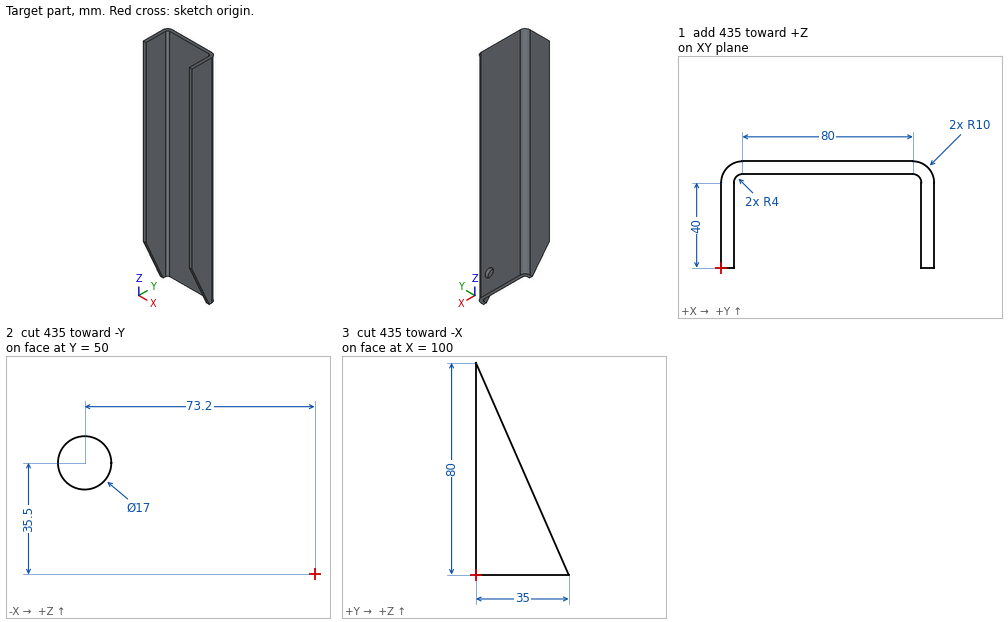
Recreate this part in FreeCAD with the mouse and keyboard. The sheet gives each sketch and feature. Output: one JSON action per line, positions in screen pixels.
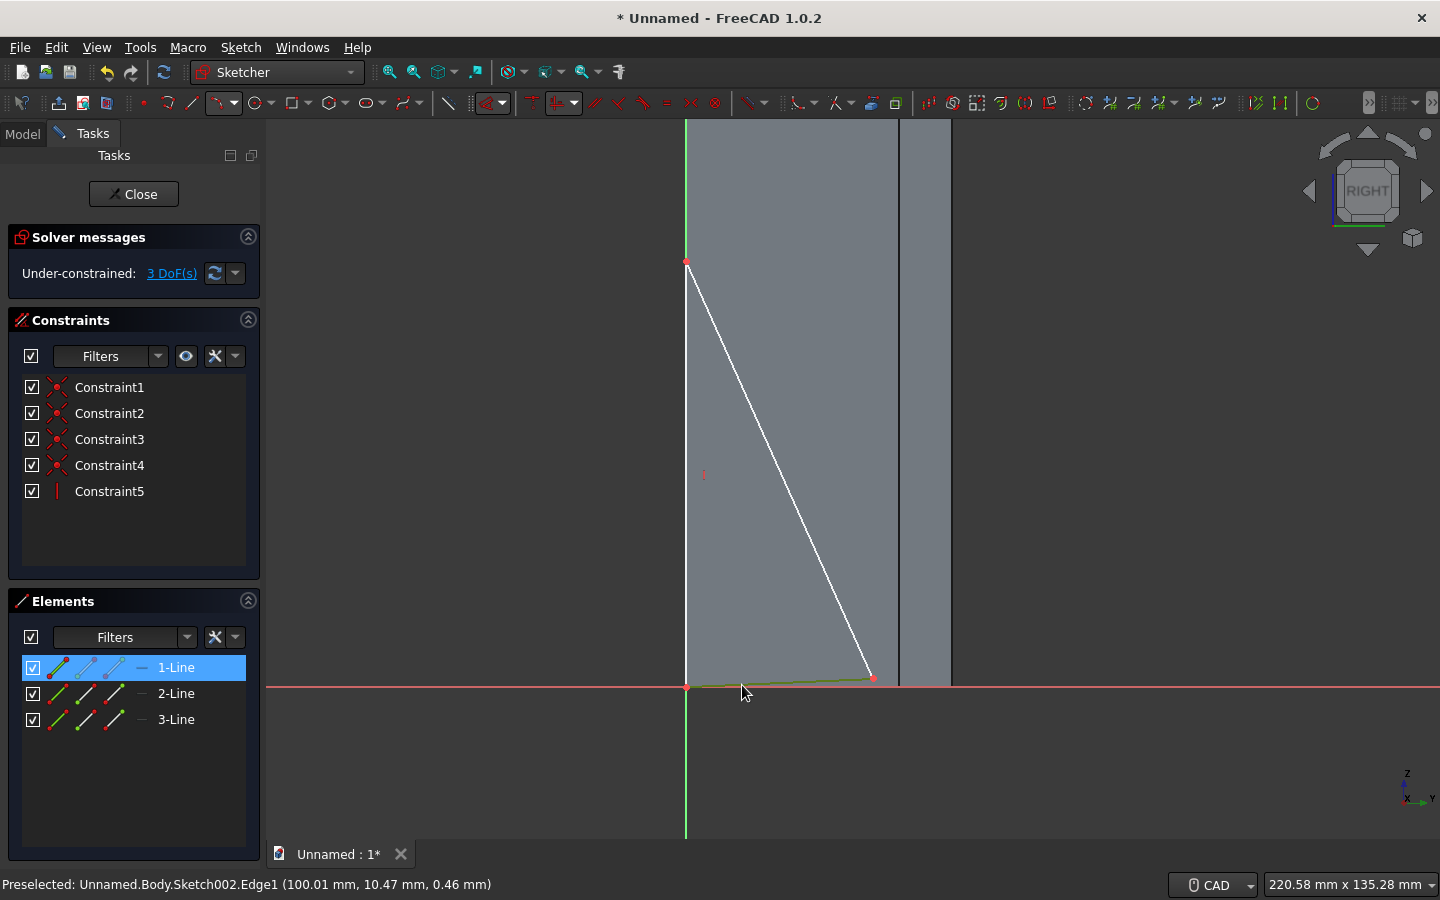
{"action": "key", "text": "h"}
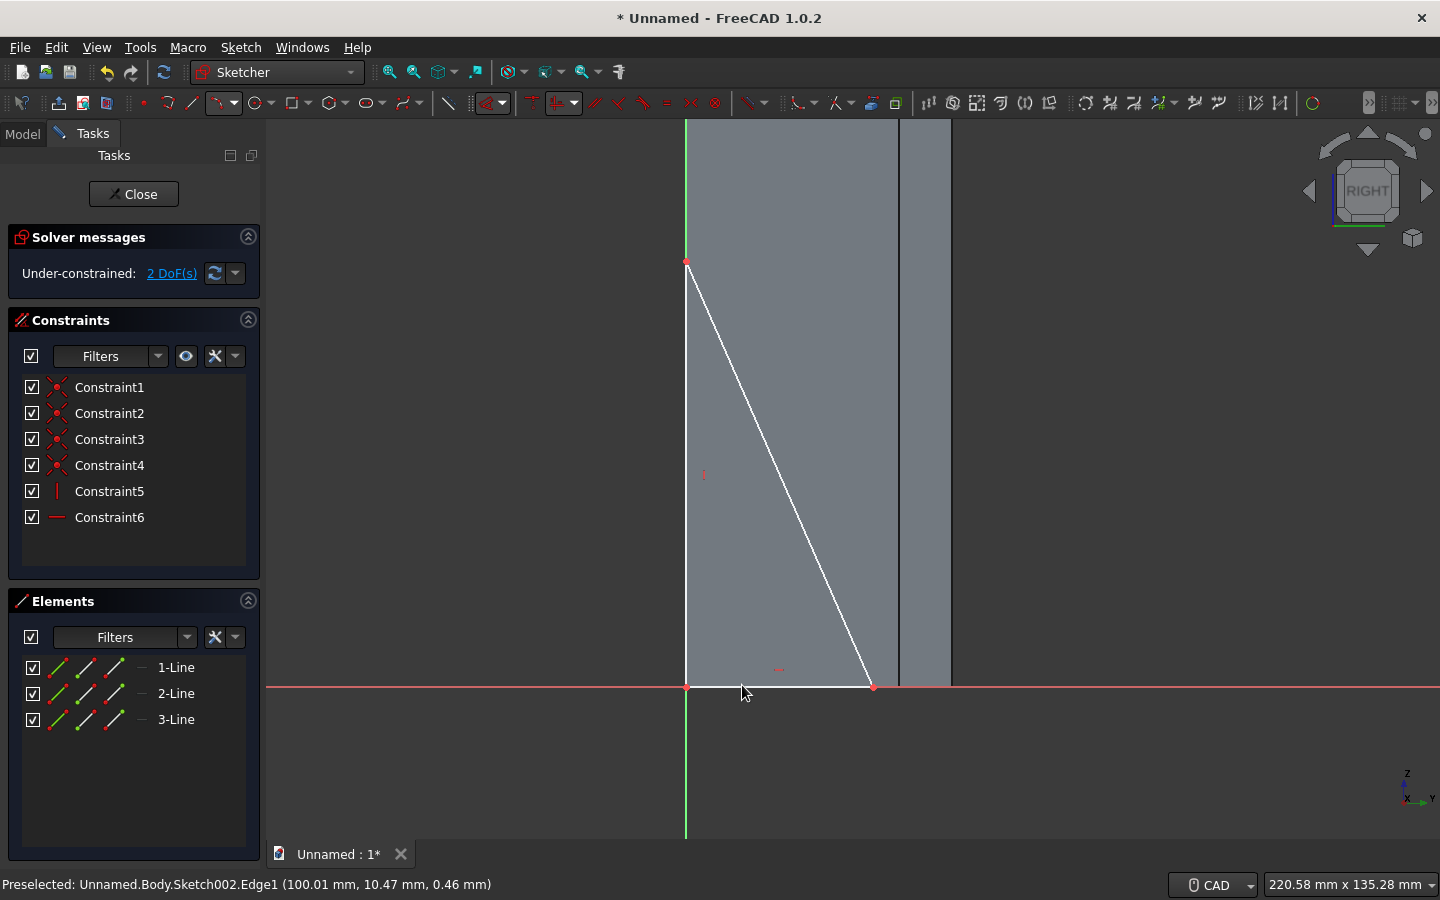
{"action": "left_click", "coordinate": [742, 687]}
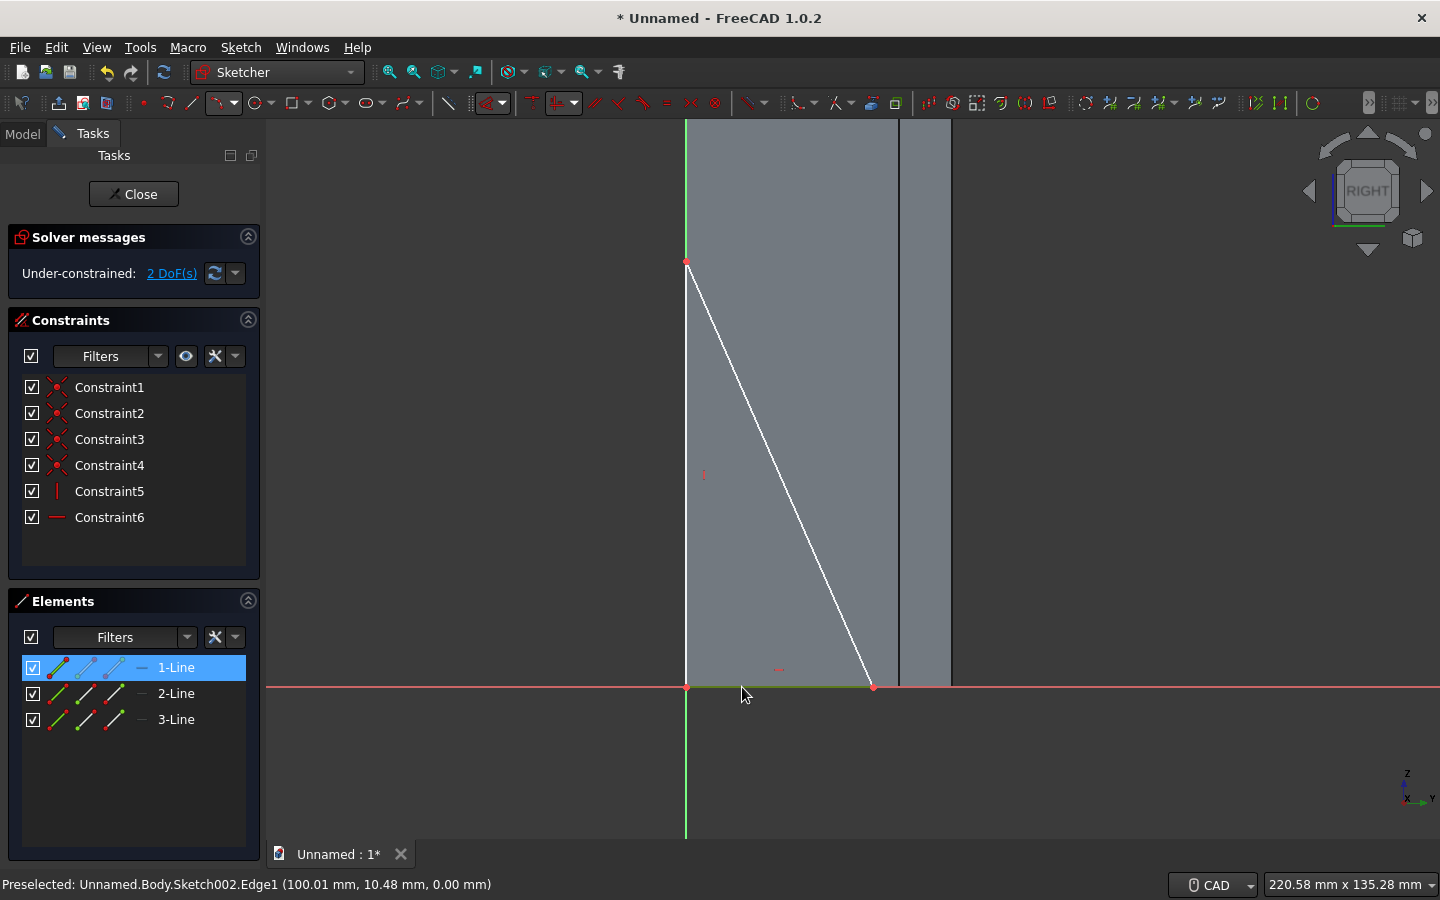
{"action": "key", "text": "l"}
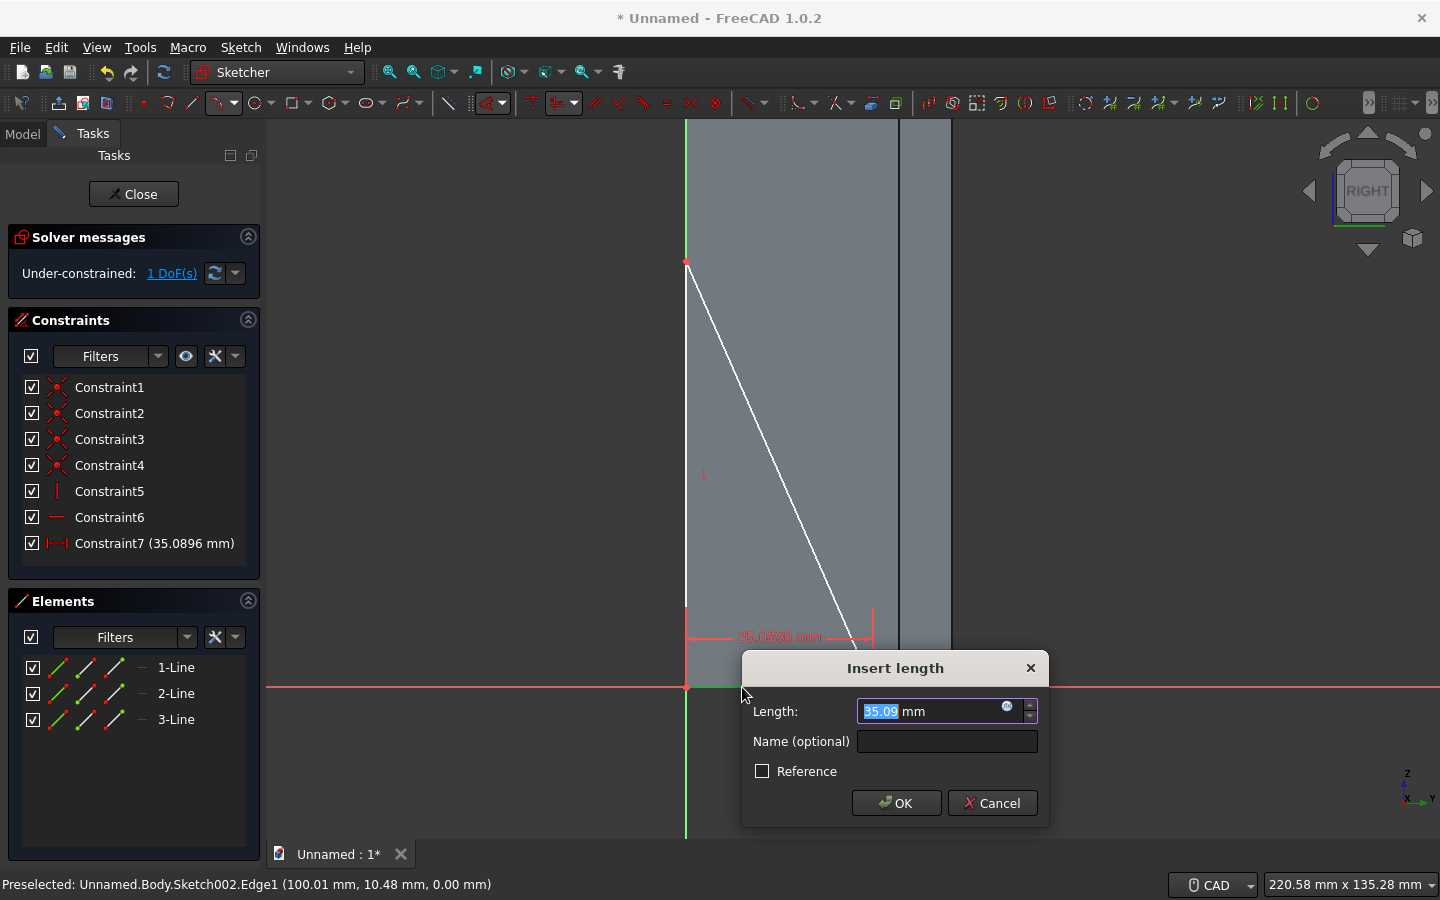
{"action": "type", "text": "35"}
{"action": "key", "text": "Return"}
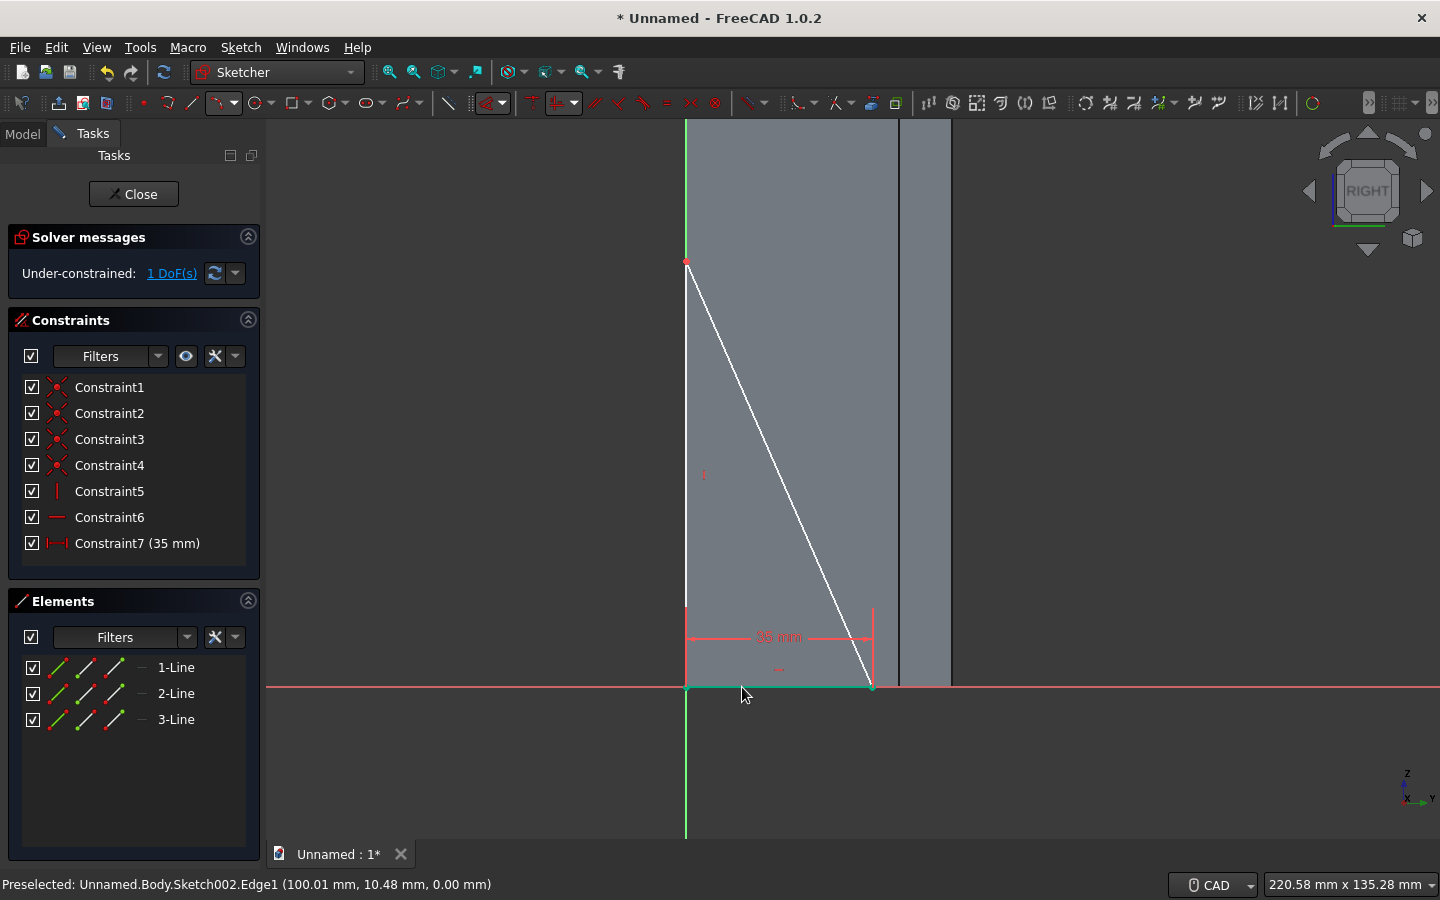
{"action": "left_click", "coordinate": [686, 390]}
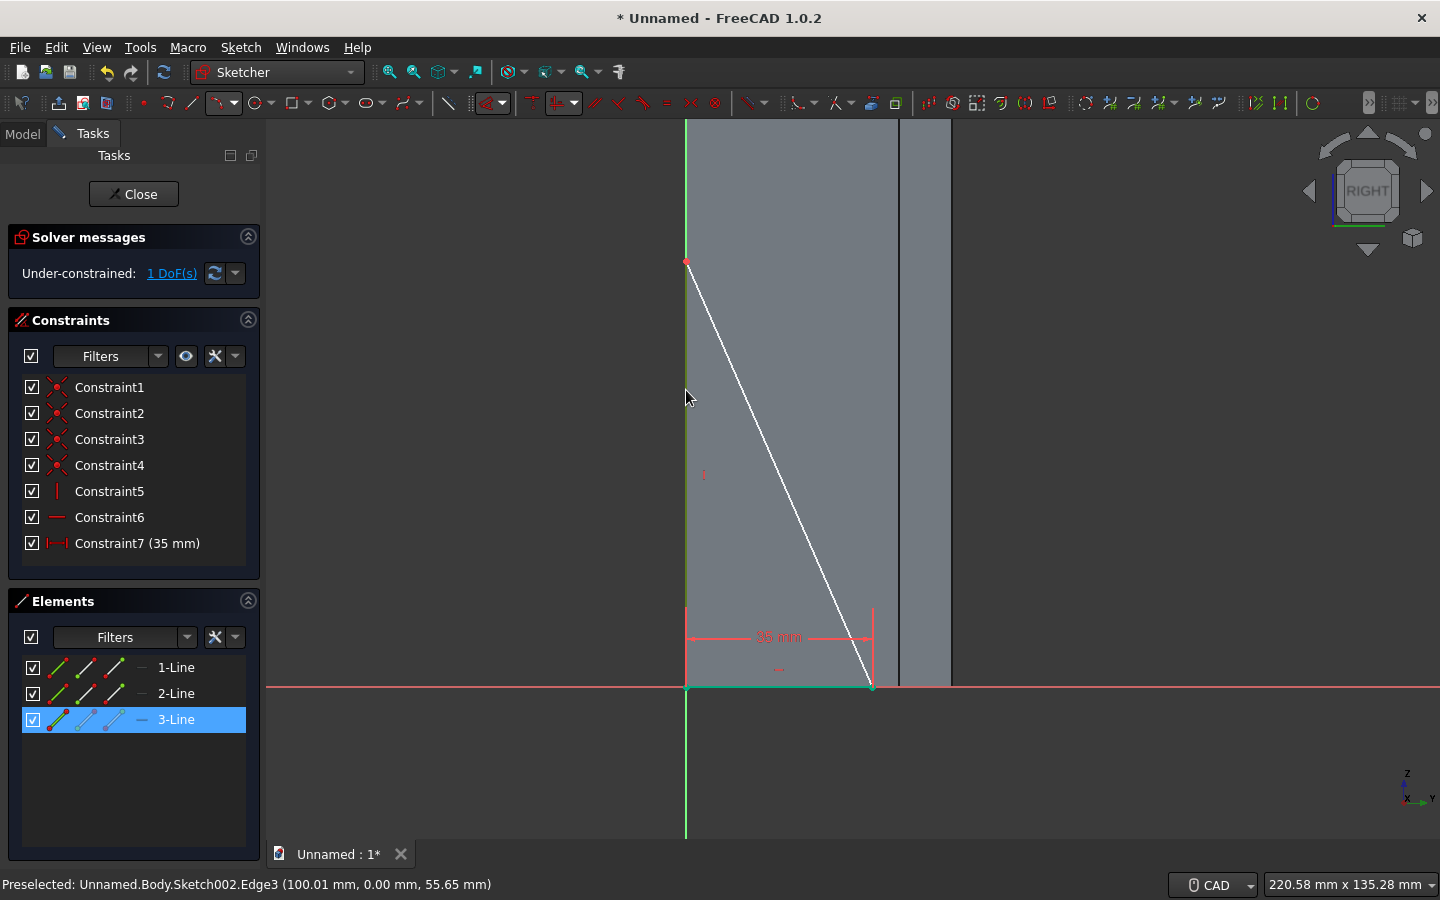
{"action": "left_click", "coordinate": [504, 104]}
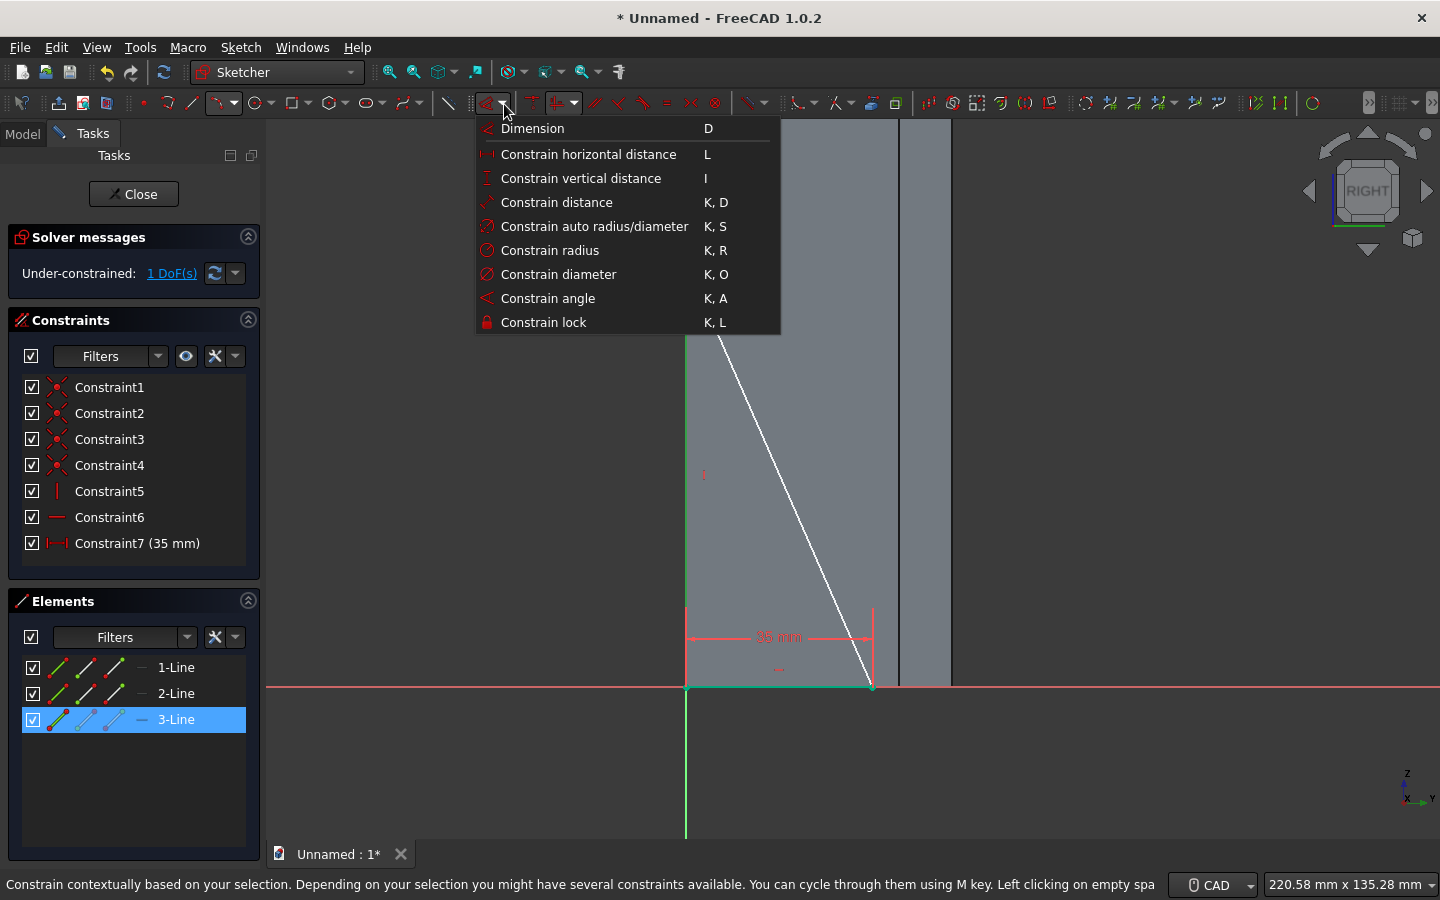
{"action": "left_click", "coordinate": [628, 178]}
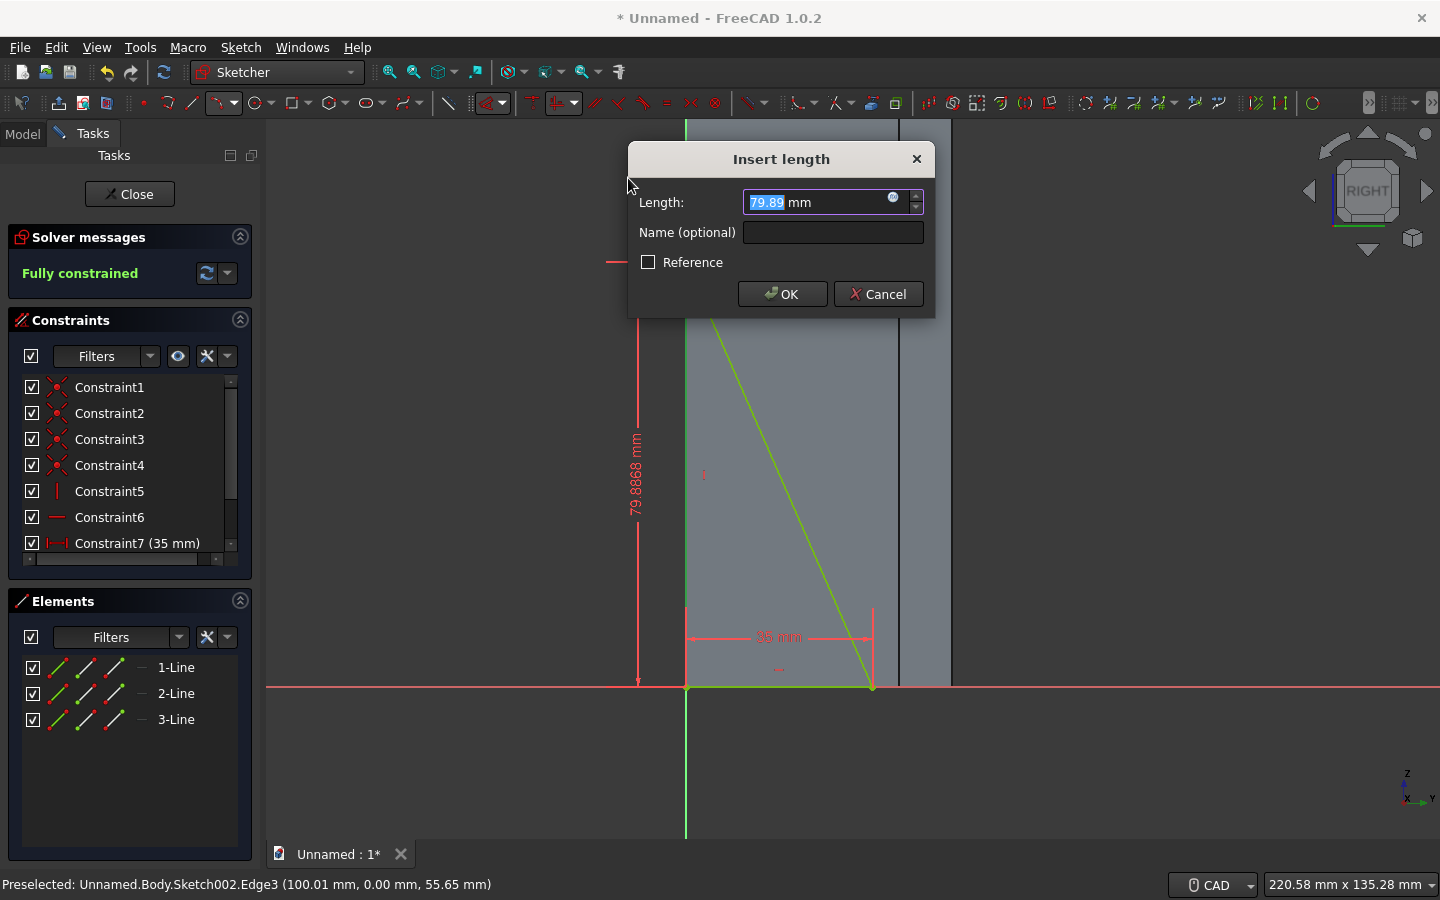
{"action": "type", "text": "80"}
{"action": "key", "text": "Return"}